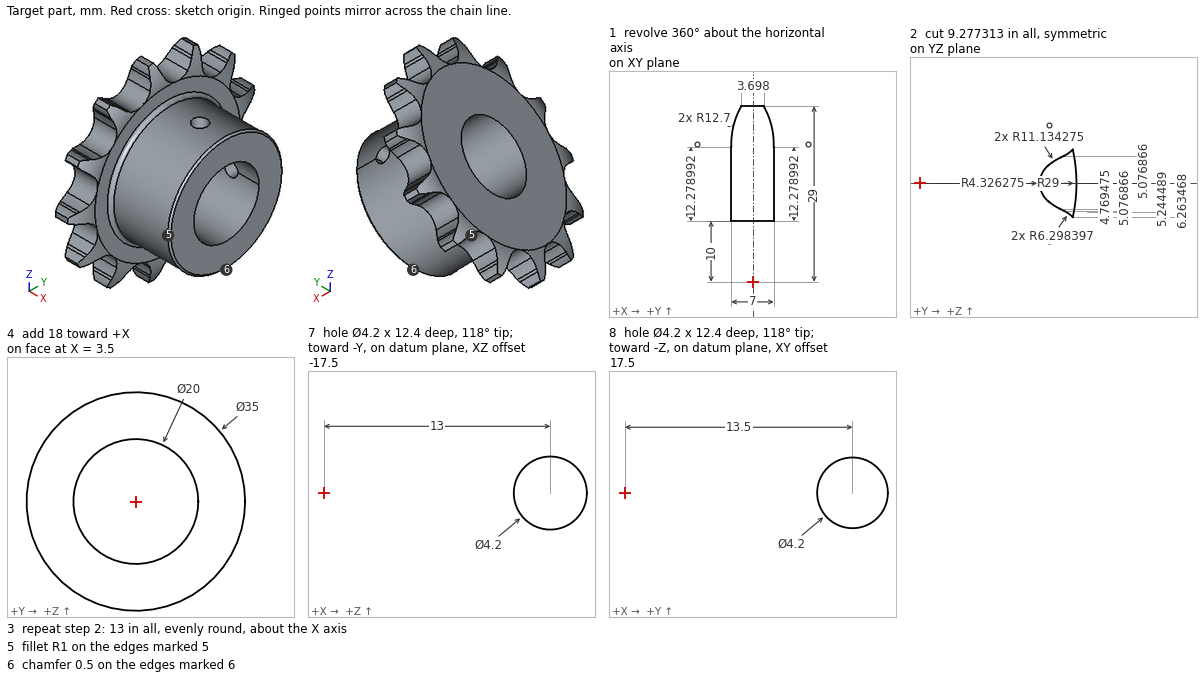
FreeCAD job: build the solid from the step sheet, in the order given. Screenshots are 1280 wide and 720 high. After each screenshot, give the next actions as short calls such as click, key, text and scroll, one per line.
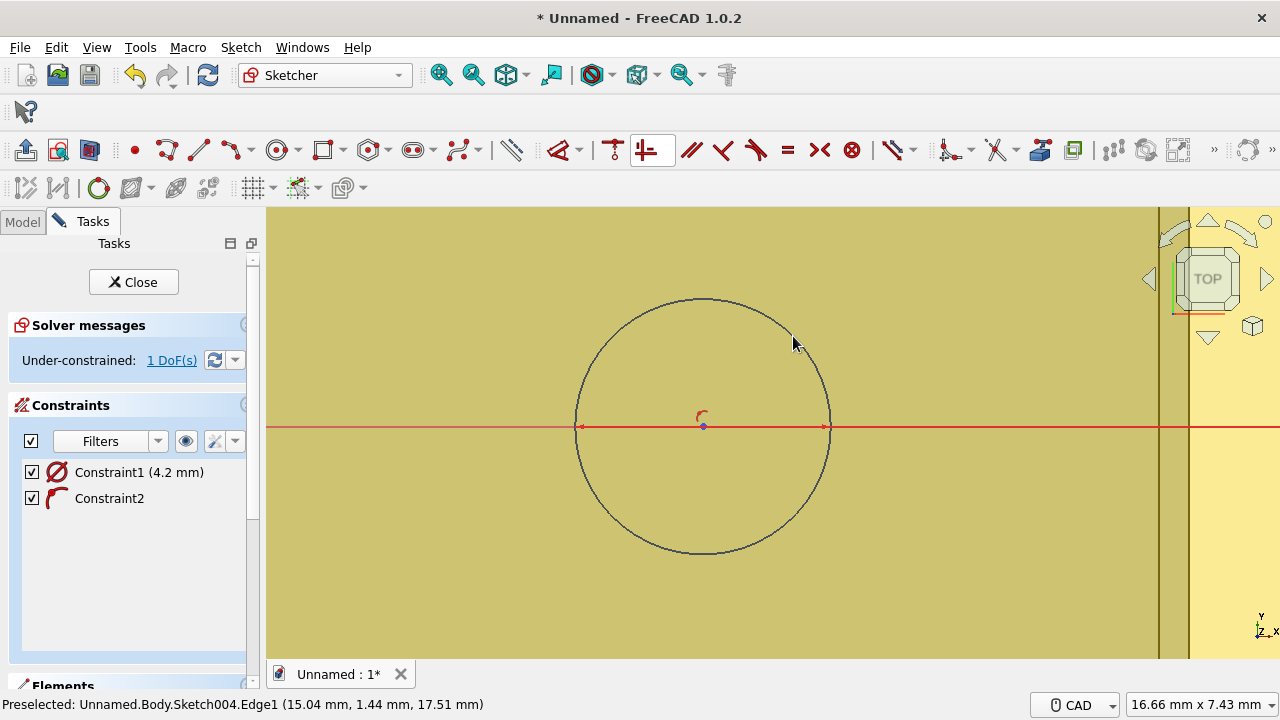
key(d)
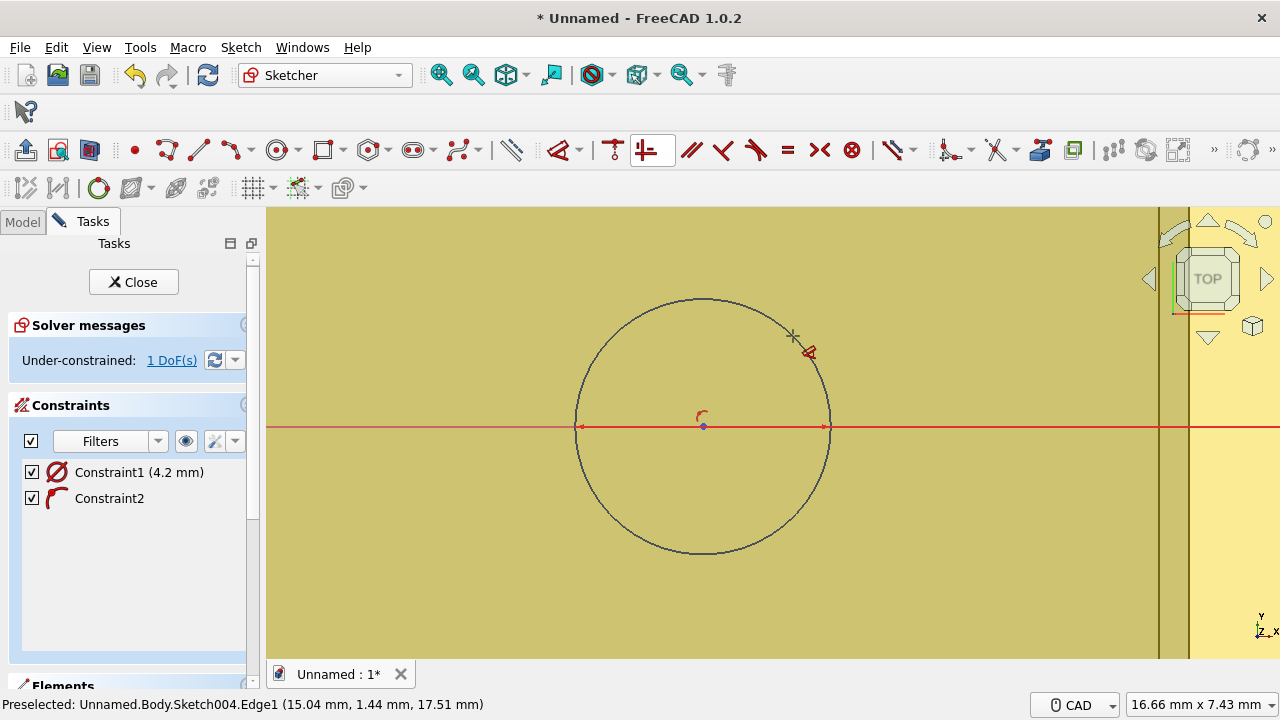
click(703, 427)
click(498, 461)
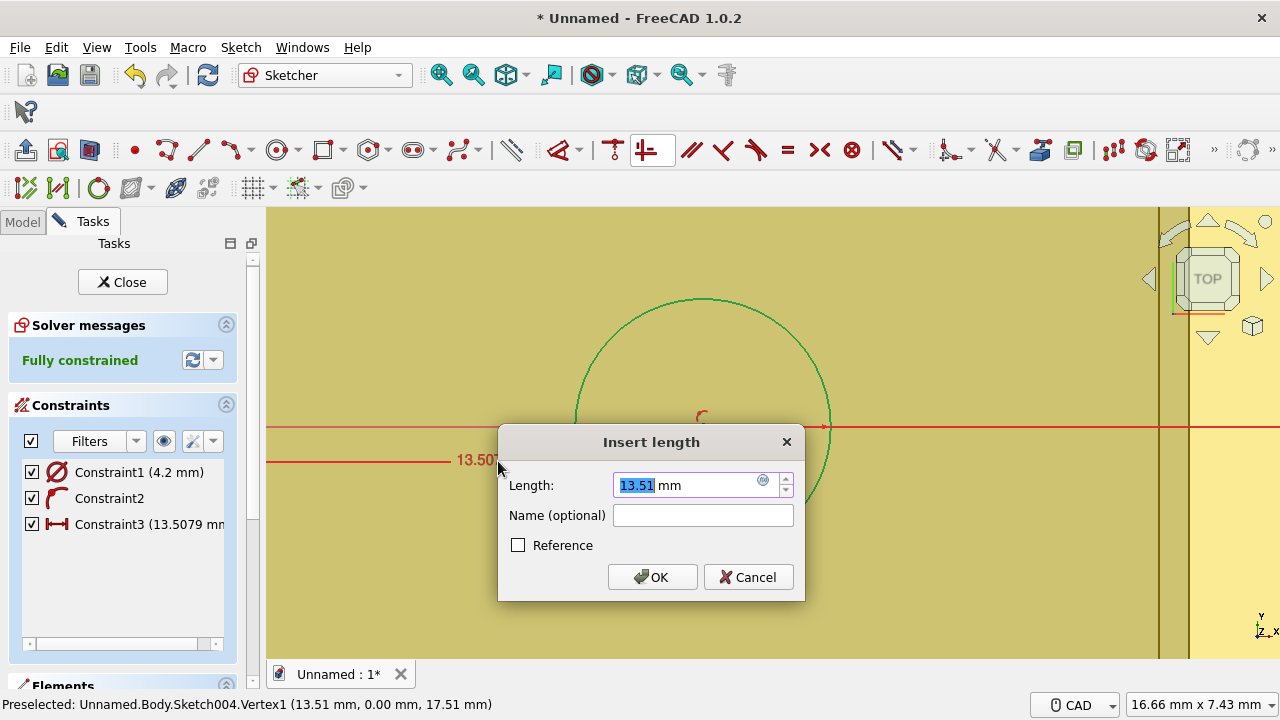
text(13.5)
key(Return)
key(Escape)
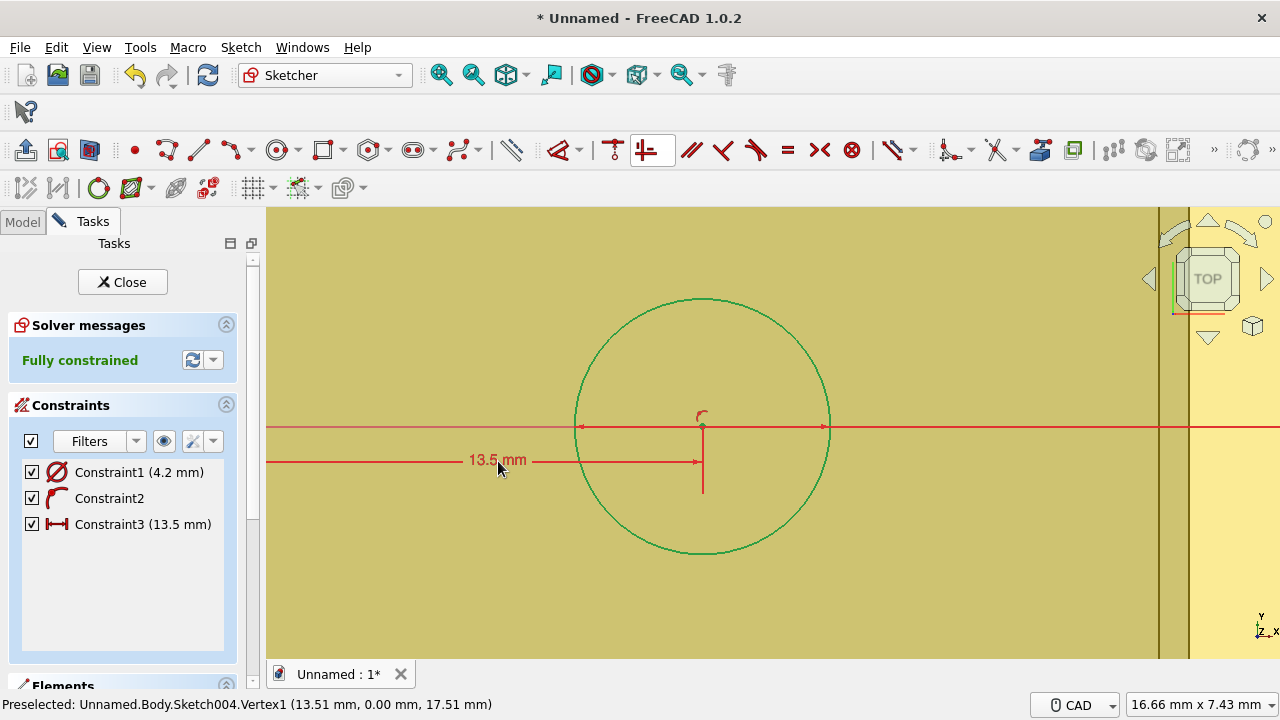
click(123, 282)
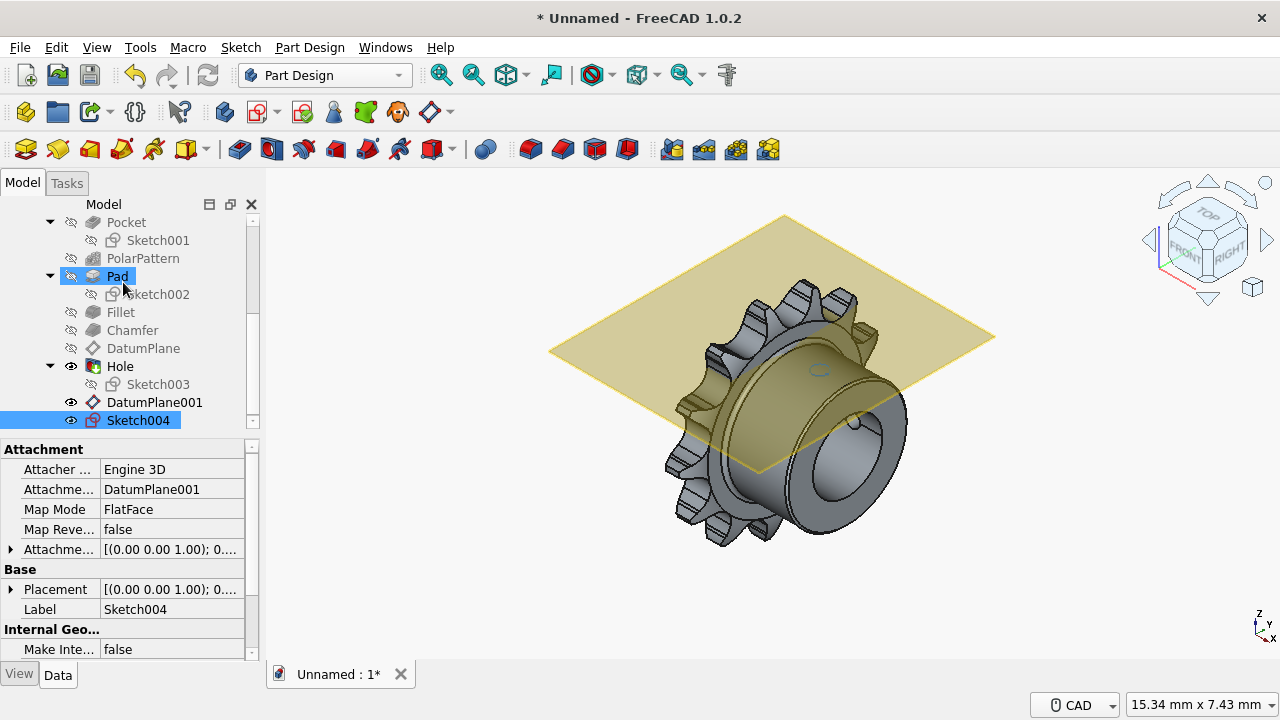
click(272, 150)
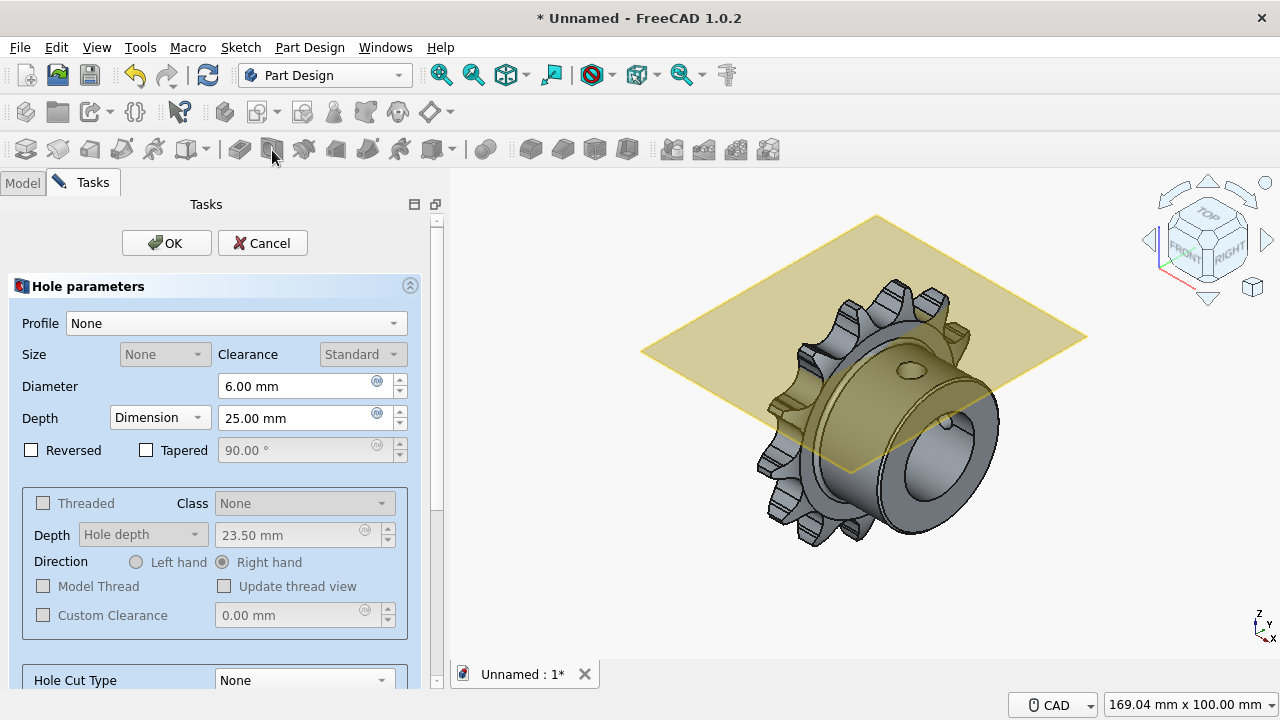
triple_click(305, 386)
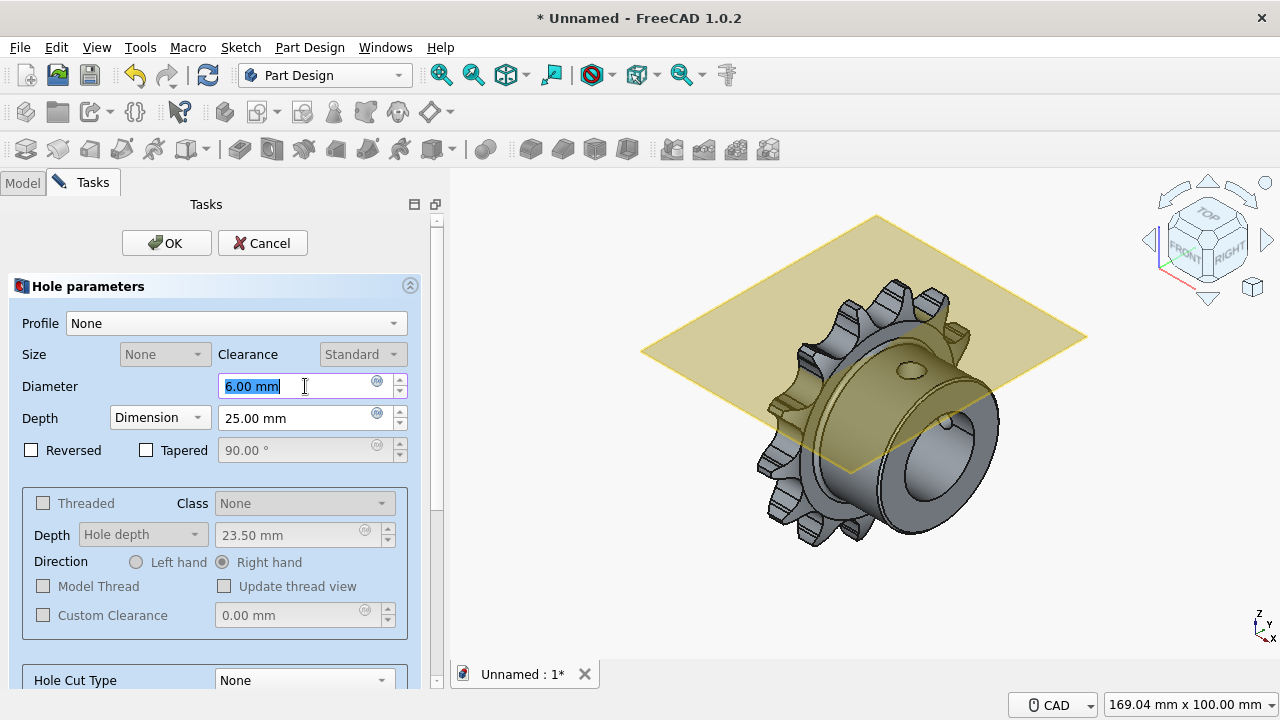
text(4.2)
key(Tab)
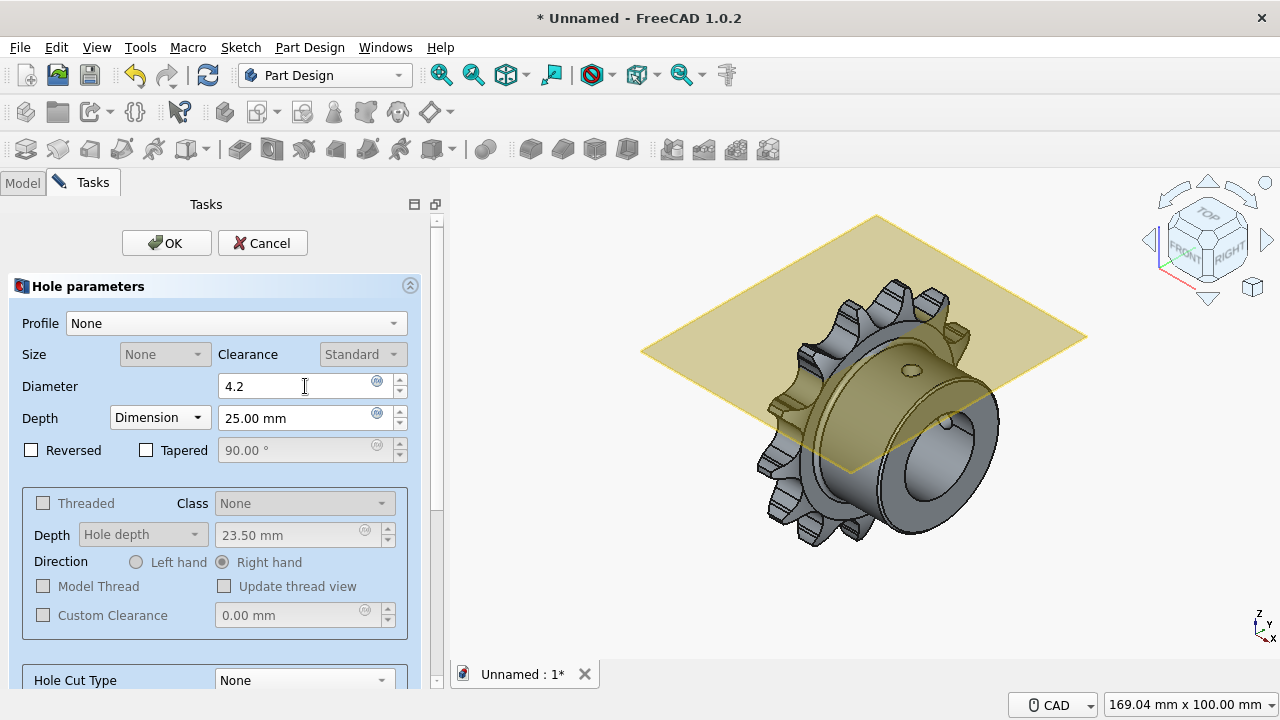
triple_click(305, 418)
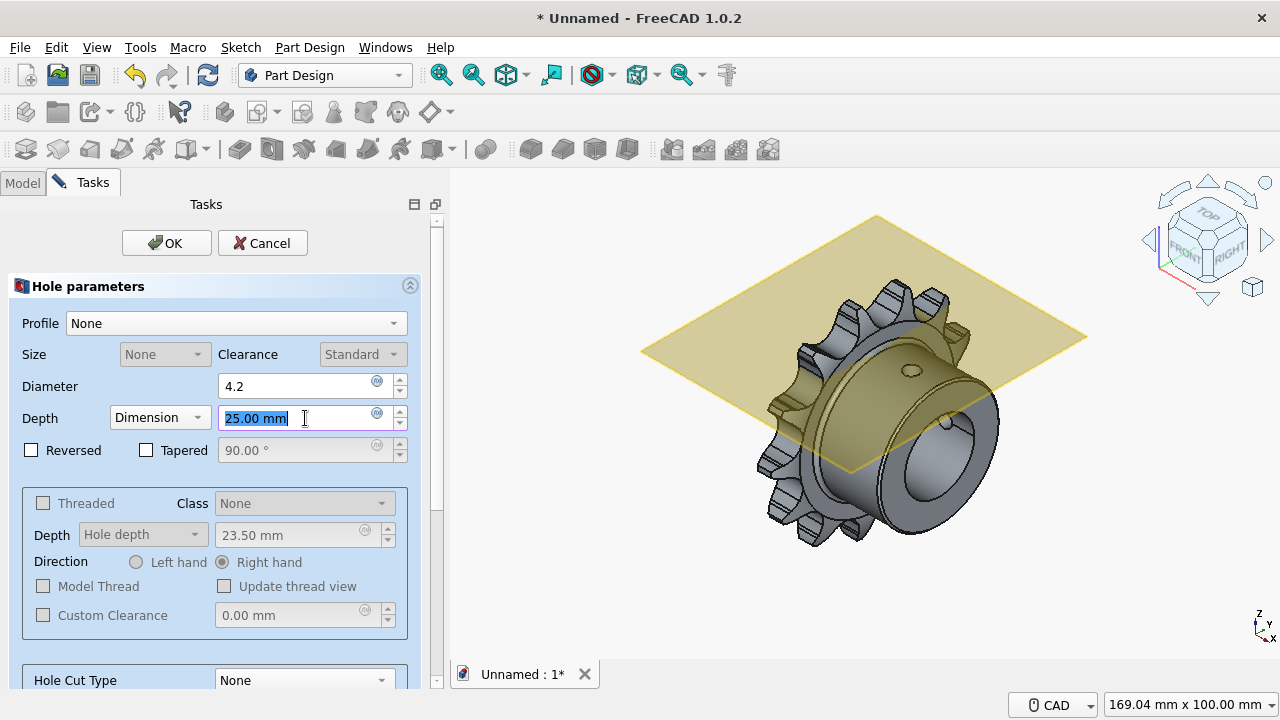
text(12.4)
key(Tab)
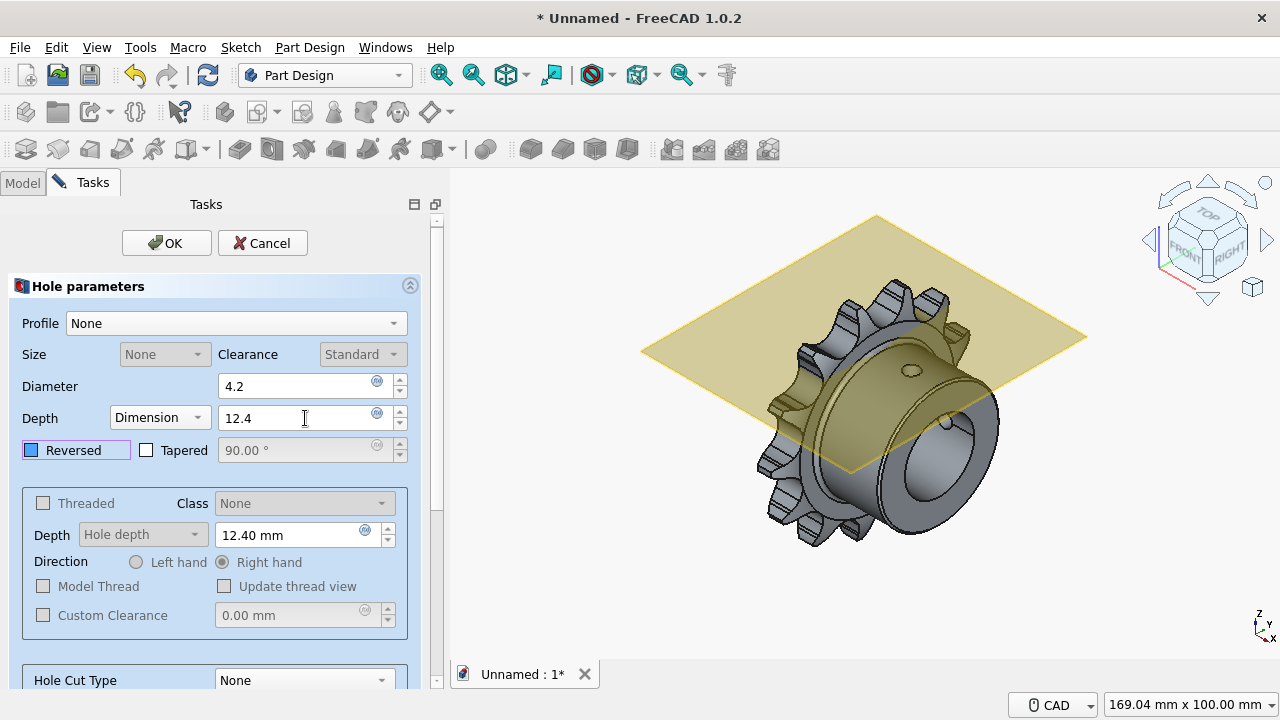
click(167, 243)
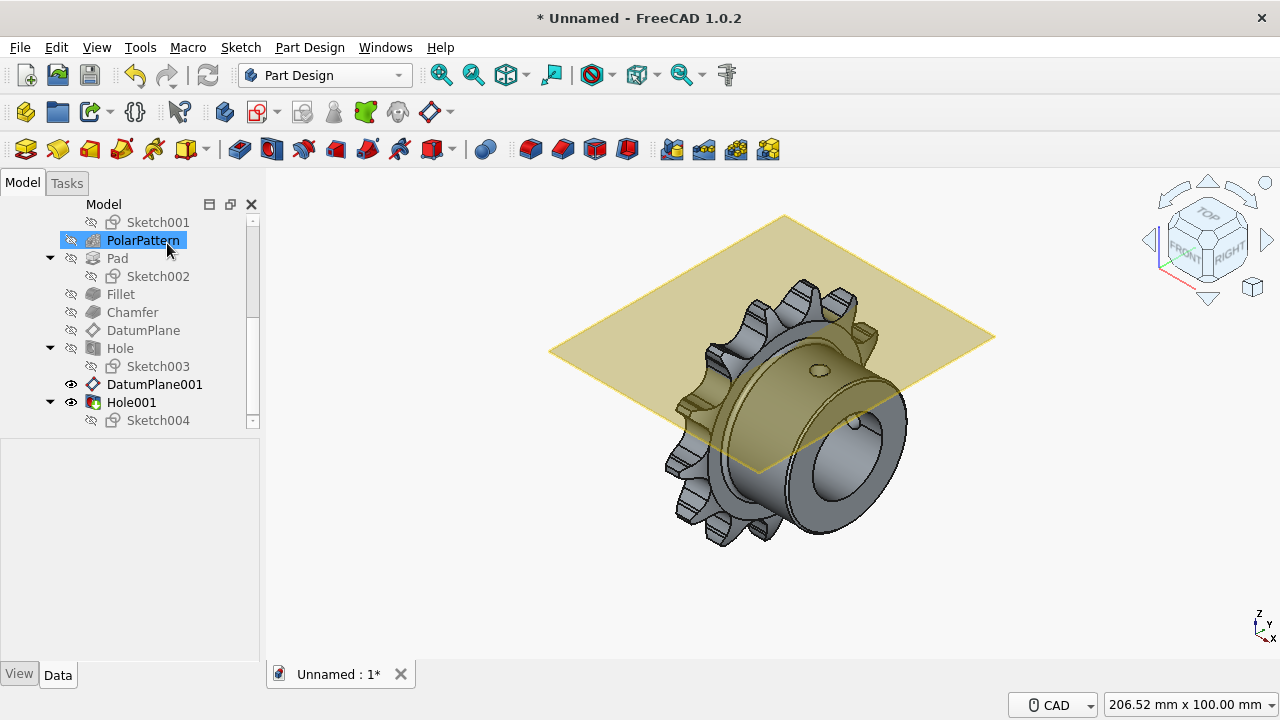
click(116, 384)
key(space)